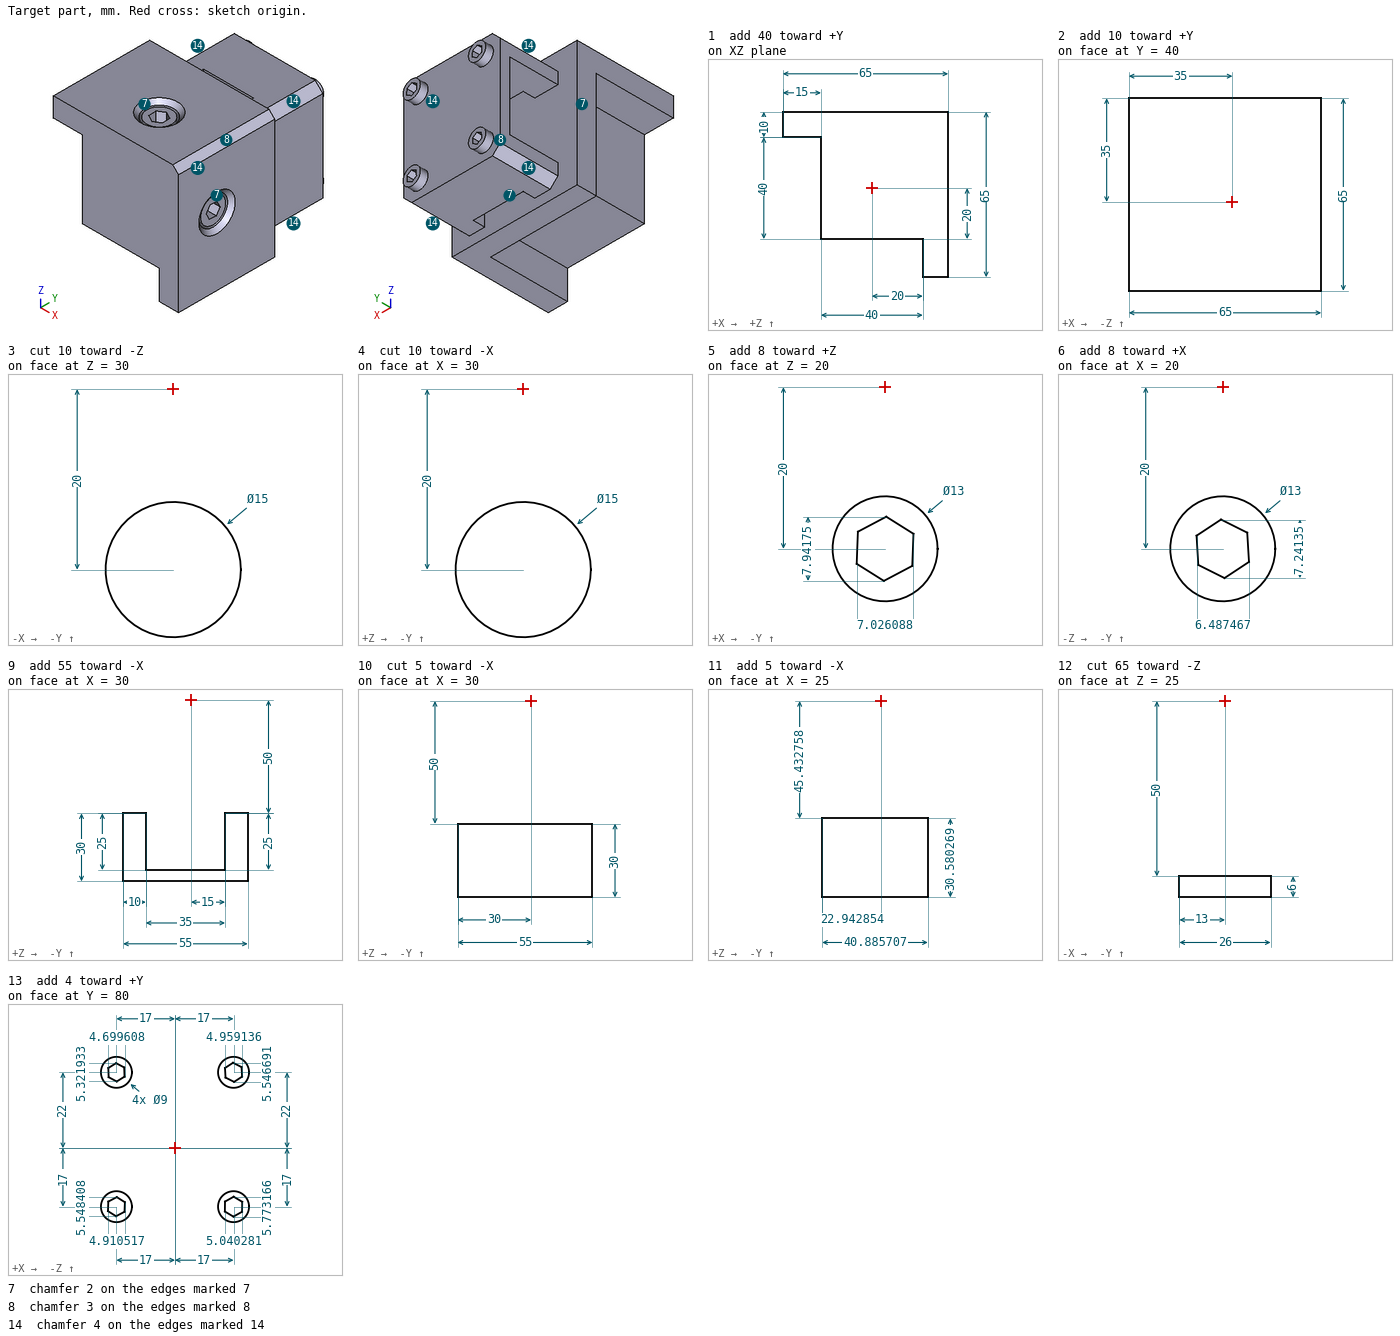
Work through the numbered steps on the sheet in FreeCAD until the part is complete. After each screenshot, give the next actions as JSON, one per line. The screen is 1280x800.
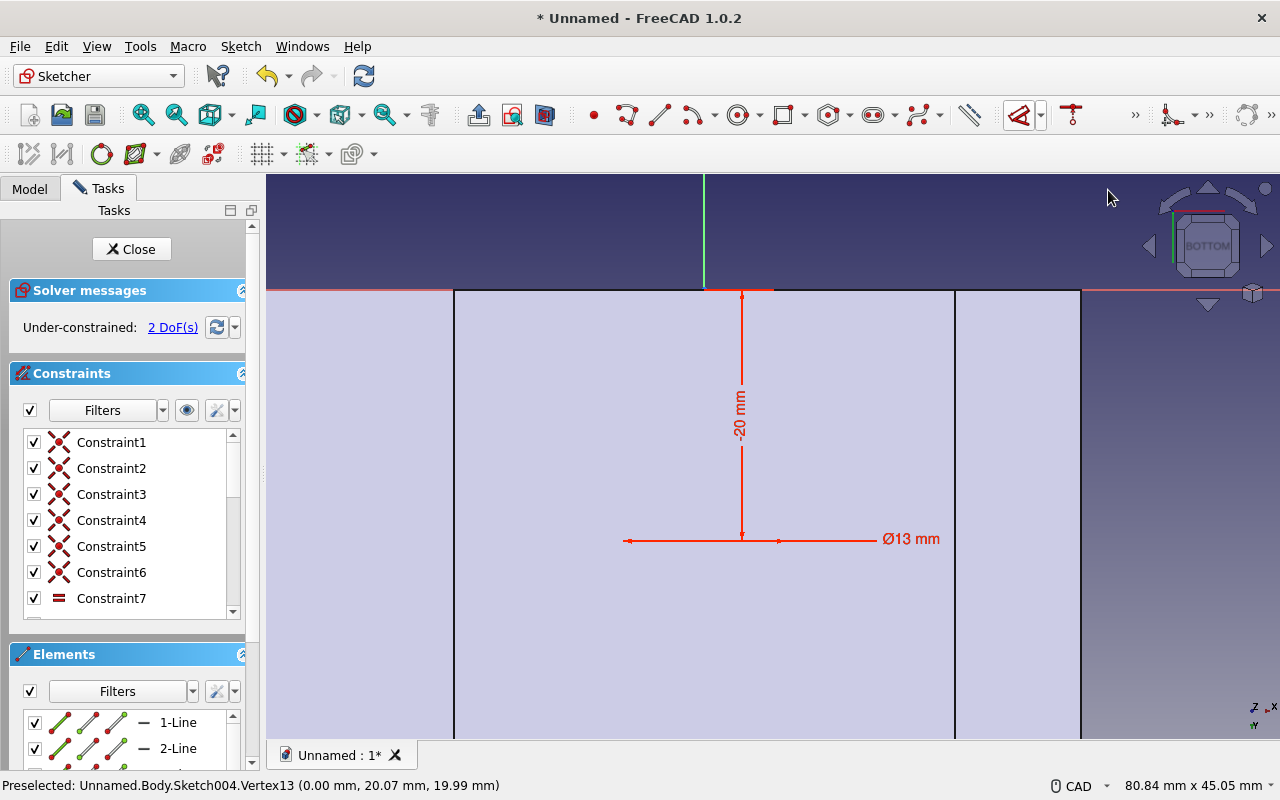
{"action": "left_click", "coordinate": [662, 565]}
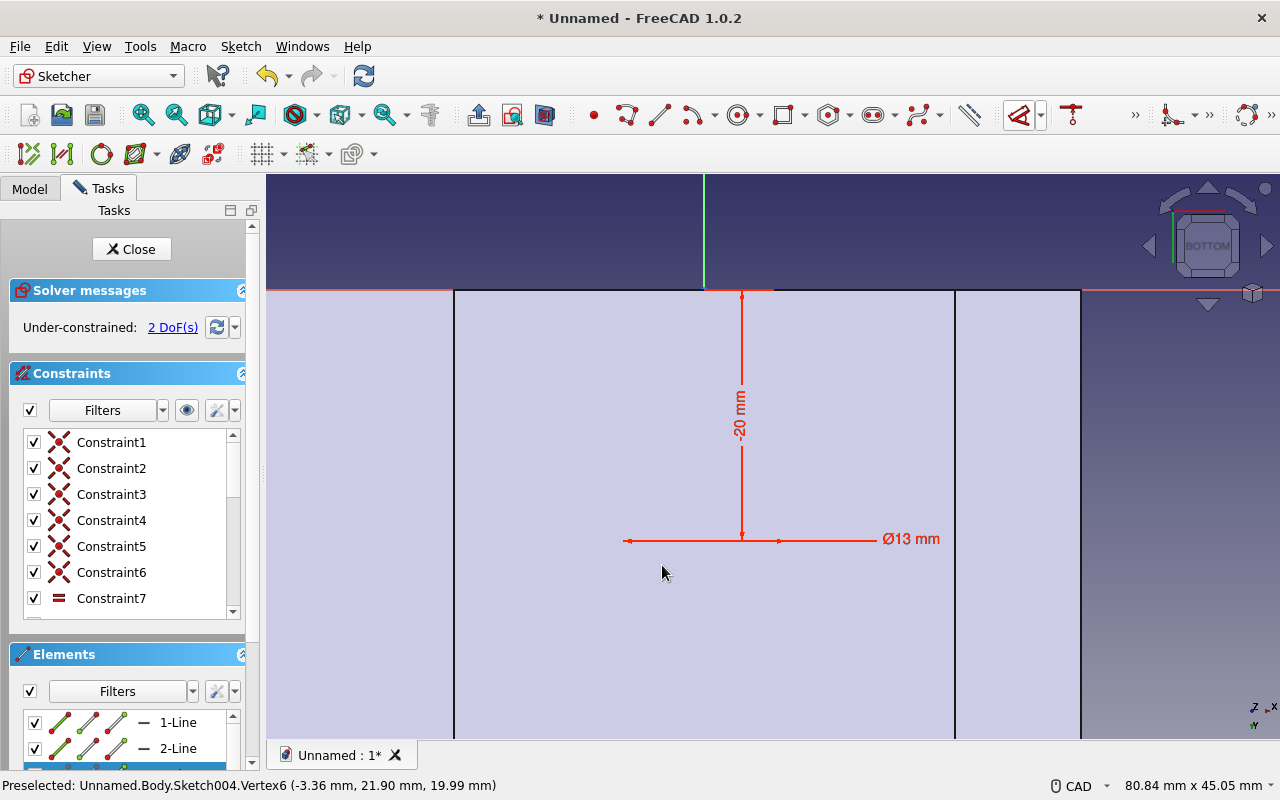
{"action": "left_click", "coordinate": [746, 517]}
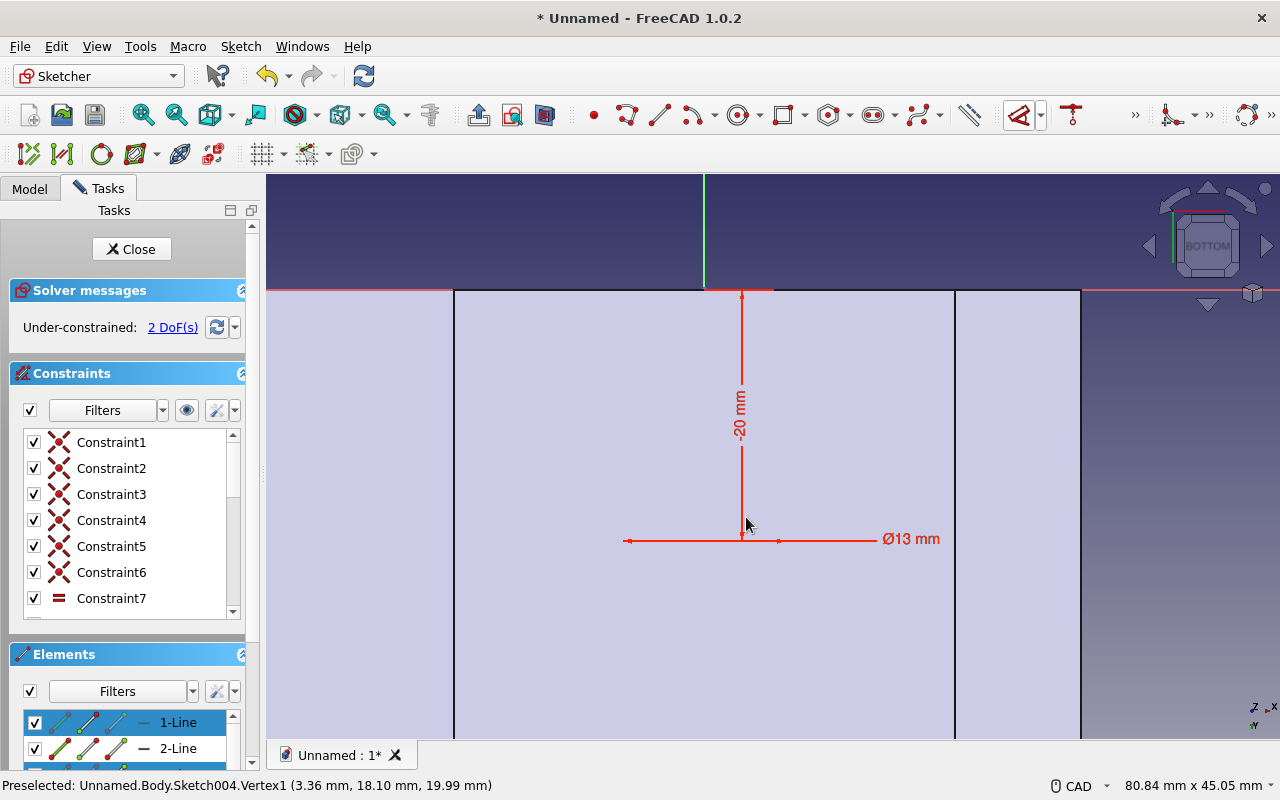
{"action": "key", "text": "l"}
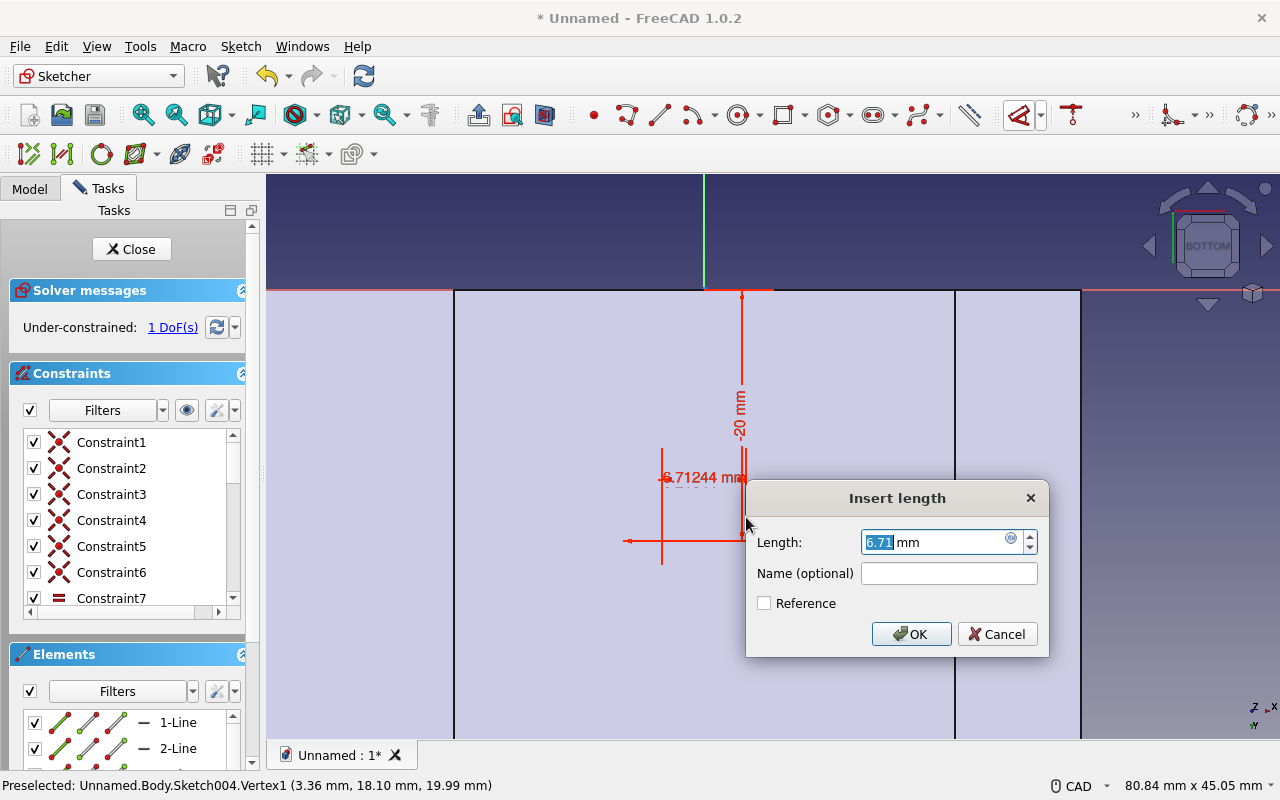
{"action": "type", "text": "7.026088"}
{"action": "key", "text": "Return"}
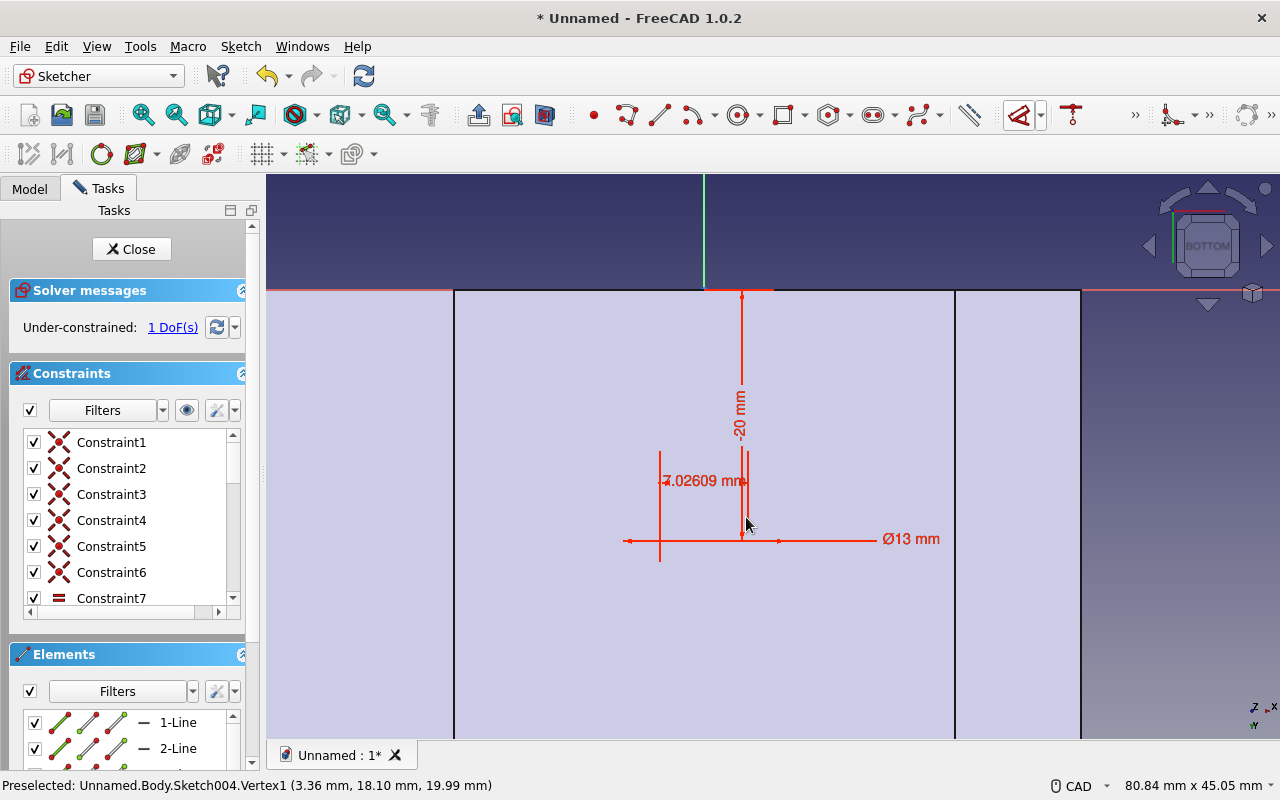
{"action": "left_click", "coordinate": [700, 590]}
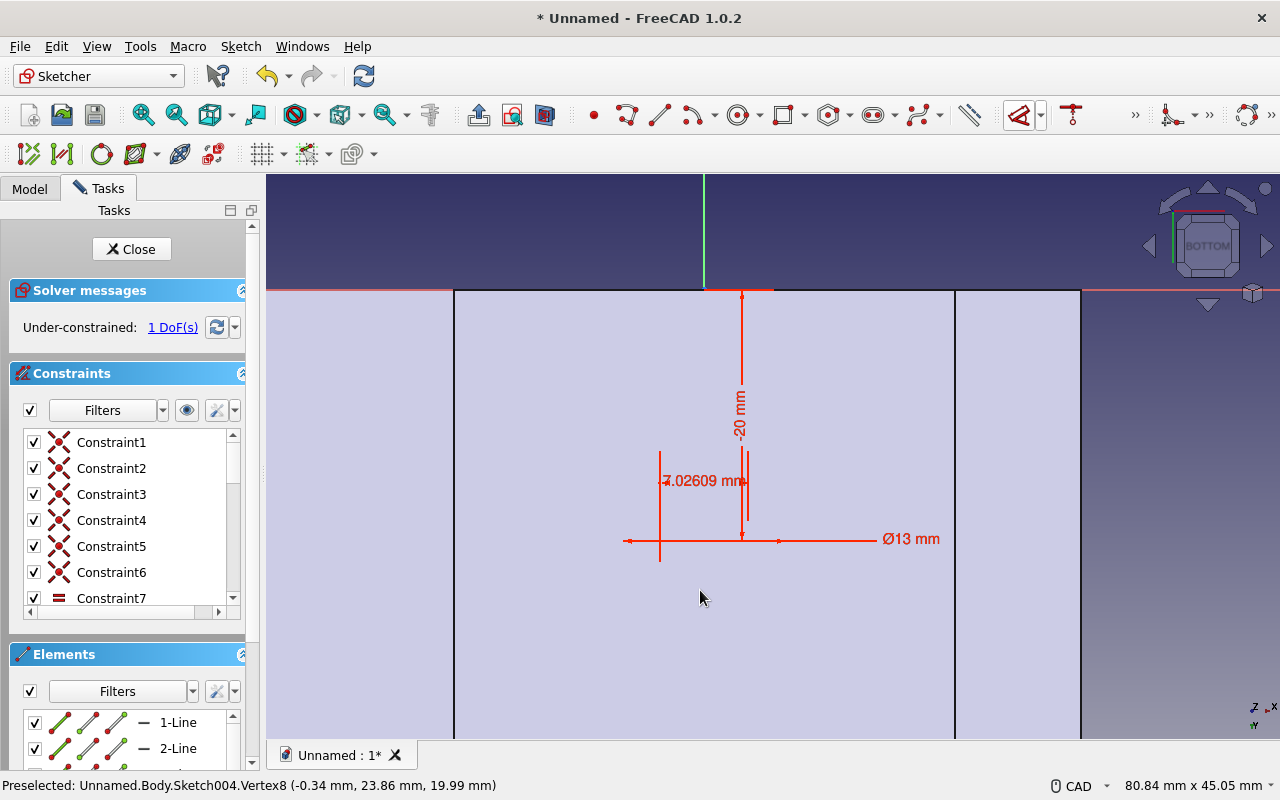
{"action": "left_click", "coordinate": [709, 493]}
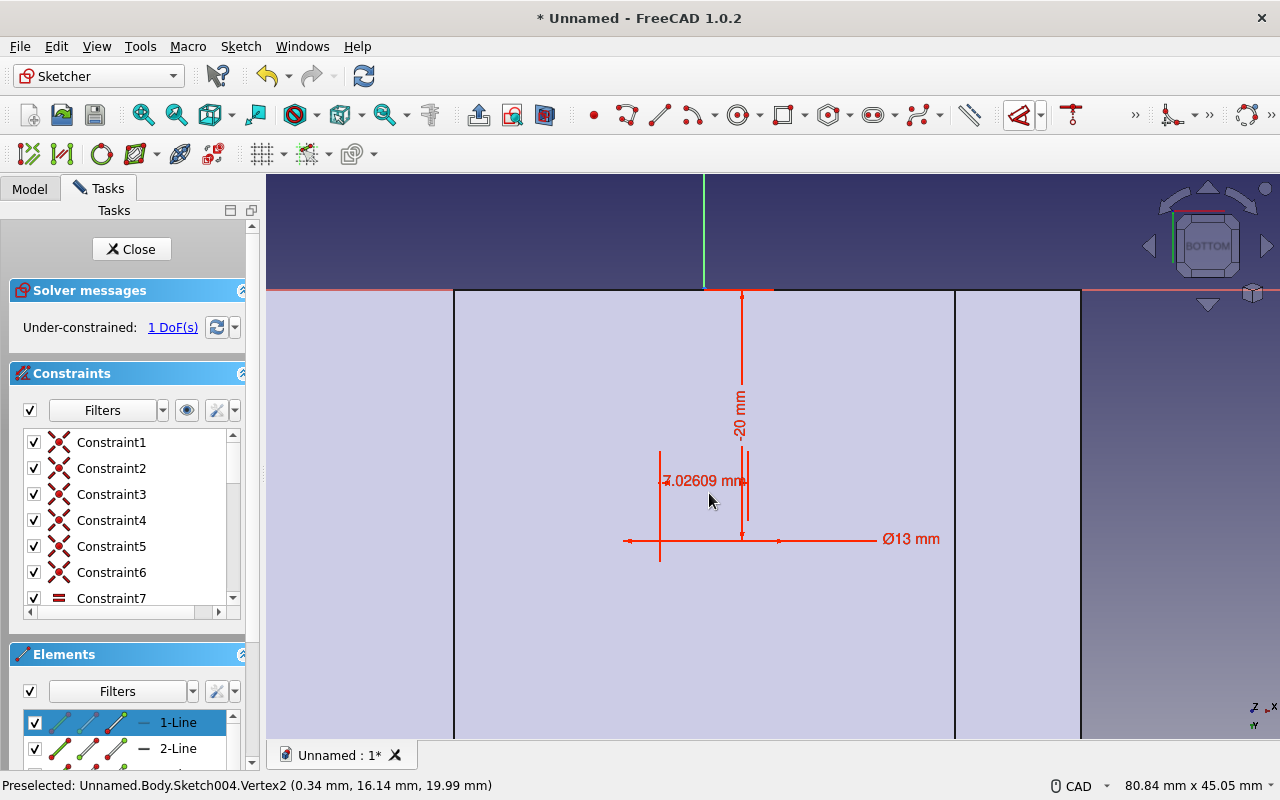
{"action": "key", "text": "i"}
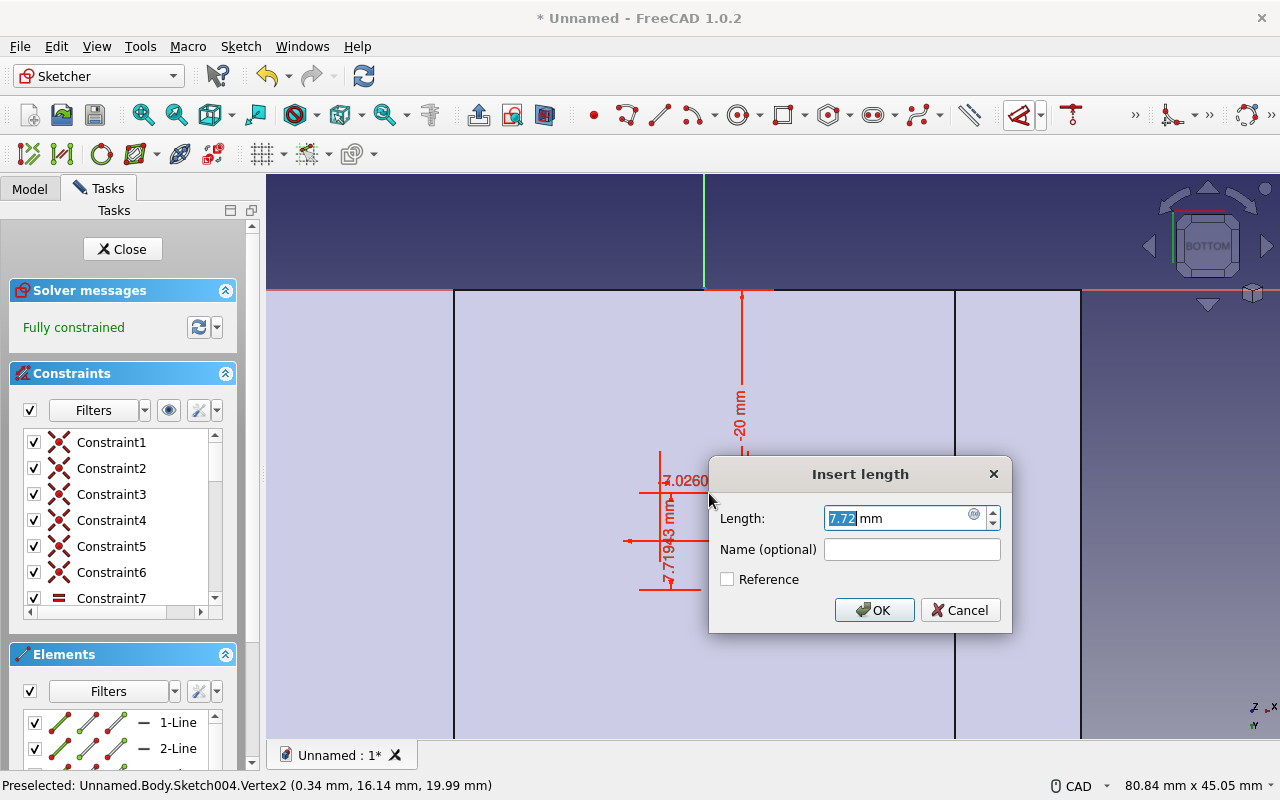
{"action": "type", "text": "7.94175"}
{"action": "key", "text": "Return"}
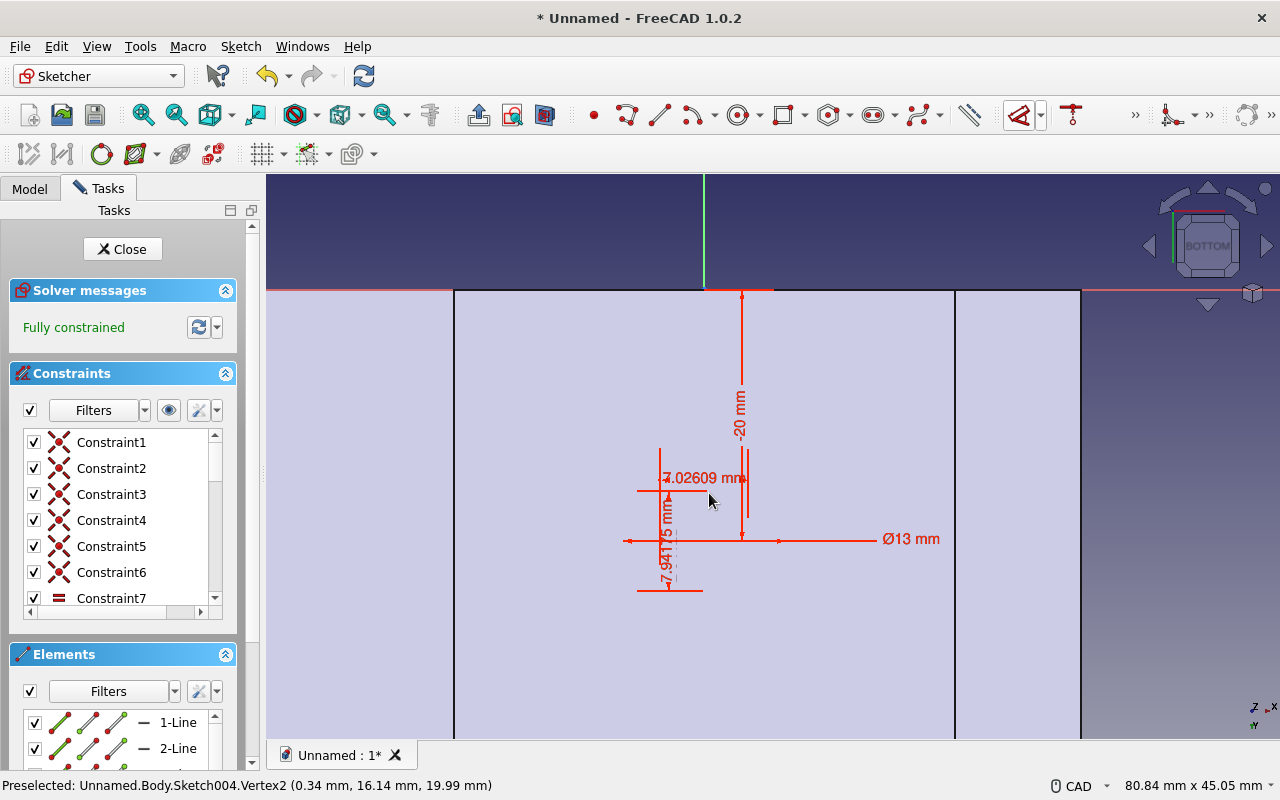
{"action": "left_click", "coordinate": [123, 249]}